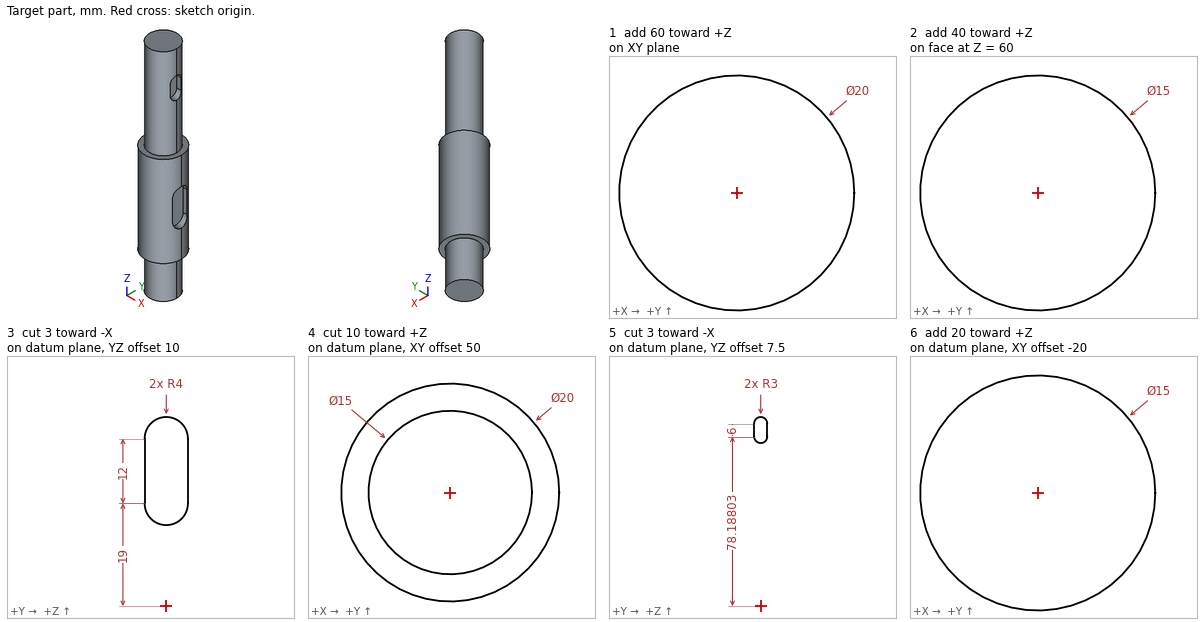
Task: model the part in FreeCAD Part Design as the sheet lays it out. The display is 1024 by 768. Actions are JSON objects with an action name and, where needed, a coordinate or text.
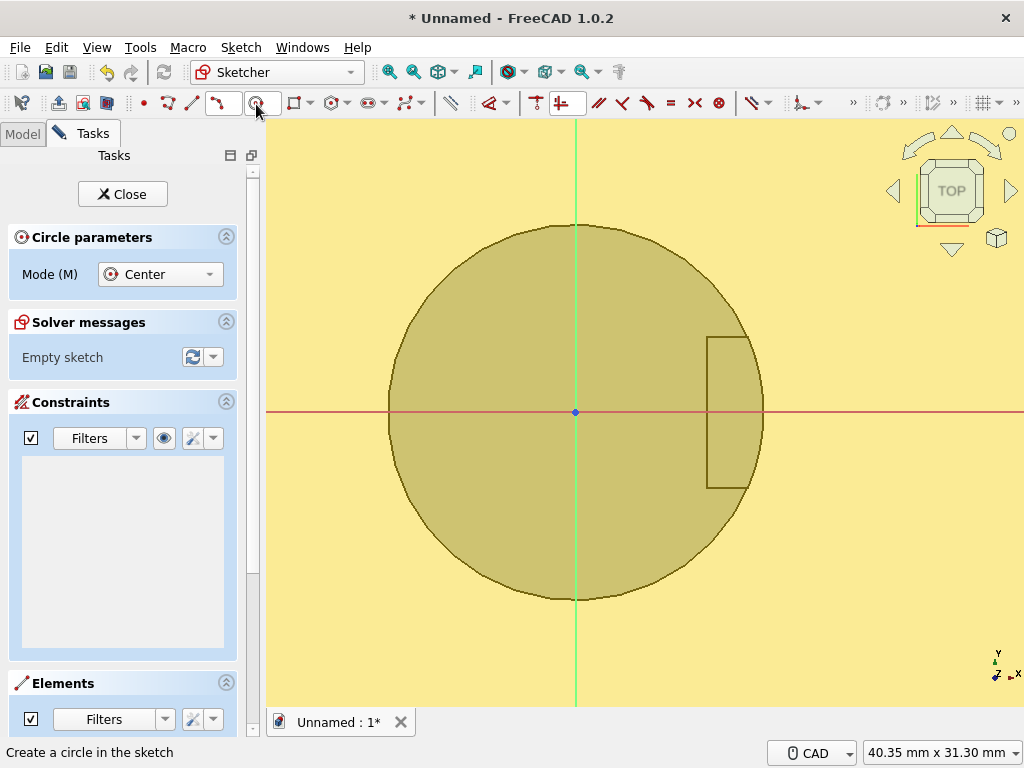
{"action": "left_click", "coordinate": [576, 412]}
{"action": "mouse_move", "coordinate": [708, 280]}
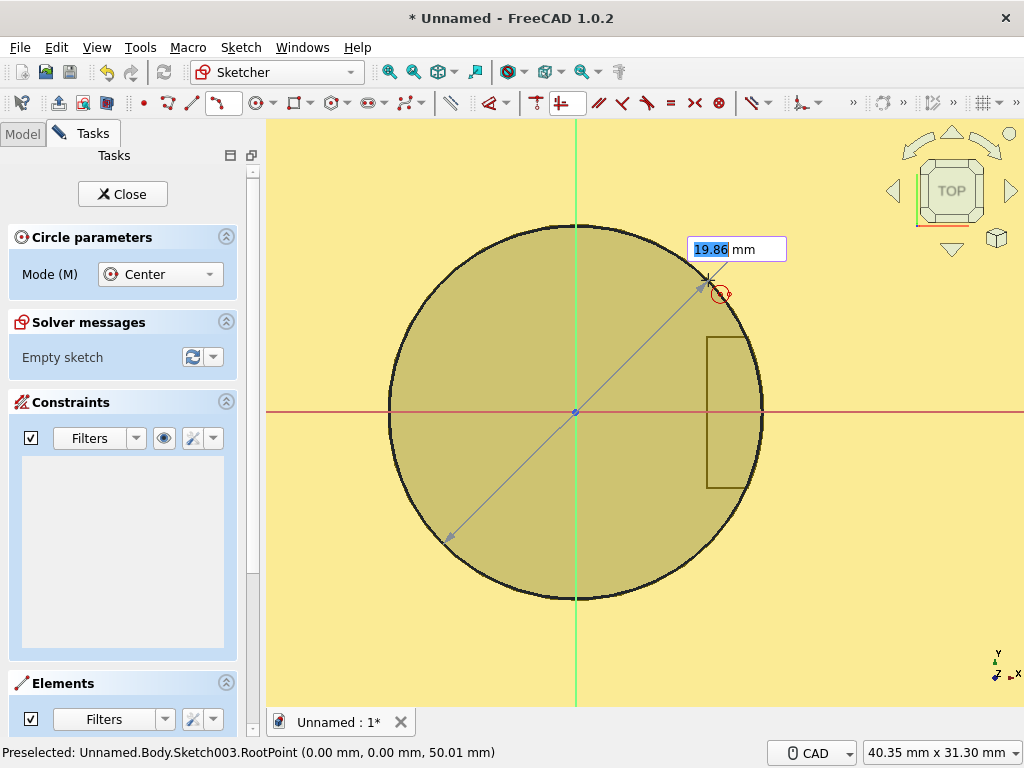
{"action": "type", "text": "20"}
{"action": "key", "text": "Return"}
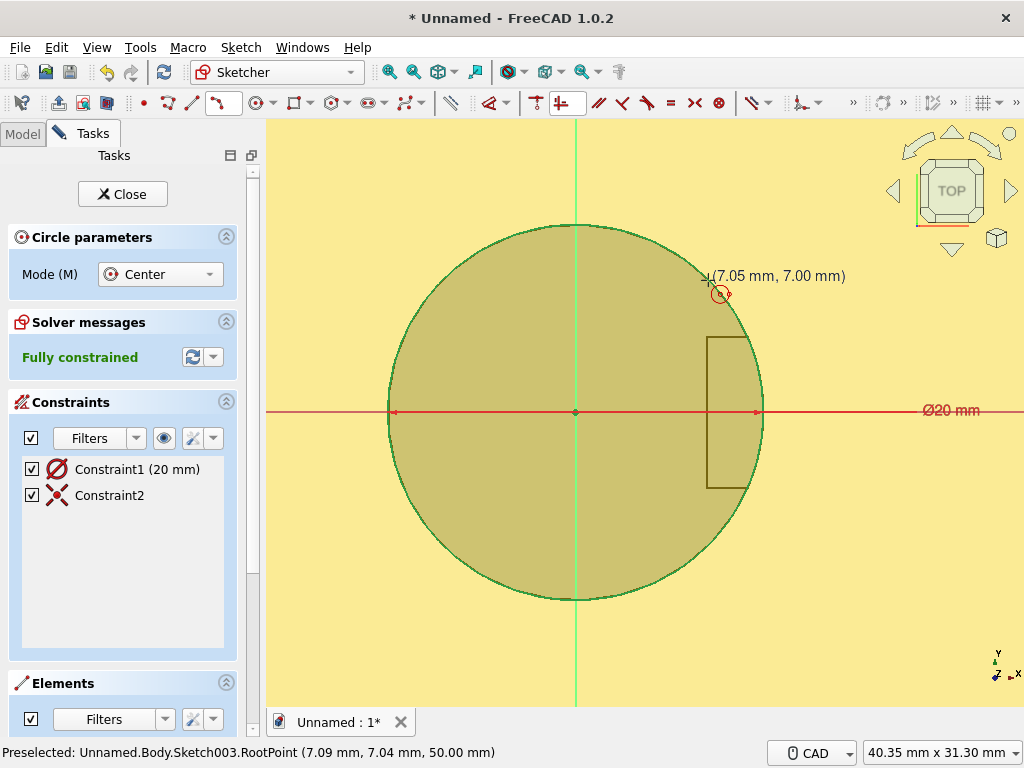
{"action": "left_click", "coordinate": [576, 412]}
{"action": "mouse_move", "coordinate": [675, 313]}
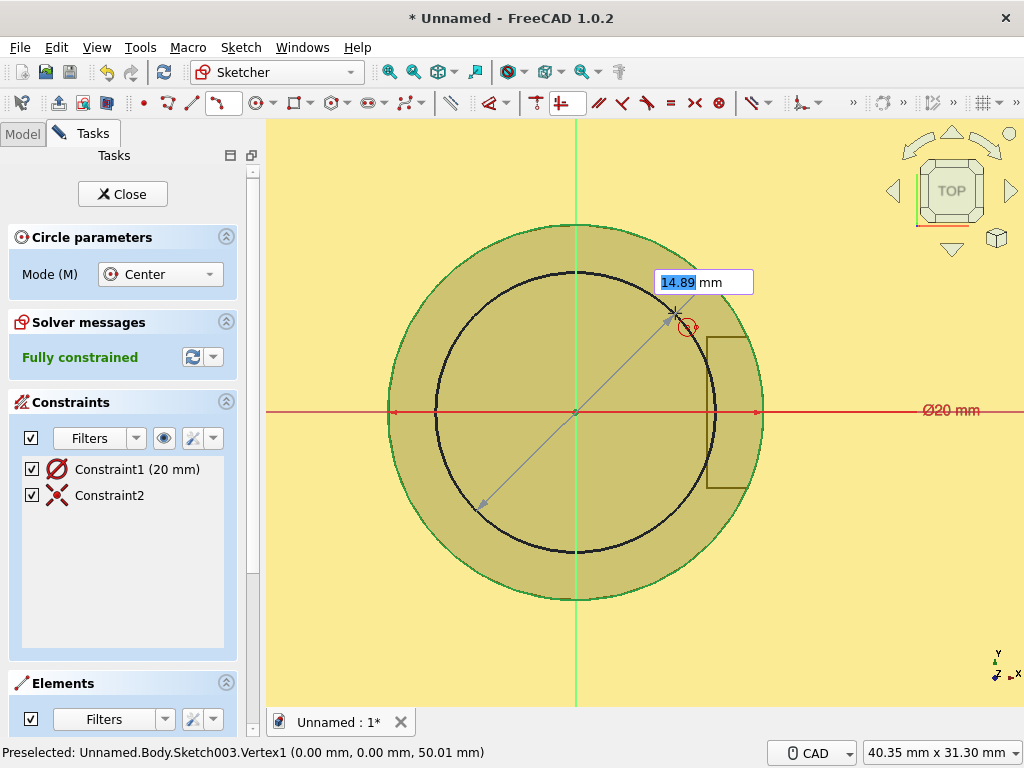
{"action": "type", "text": "15"}
{"action": "key", "text": "Return"}
{"action": "key", "text": "Escape"}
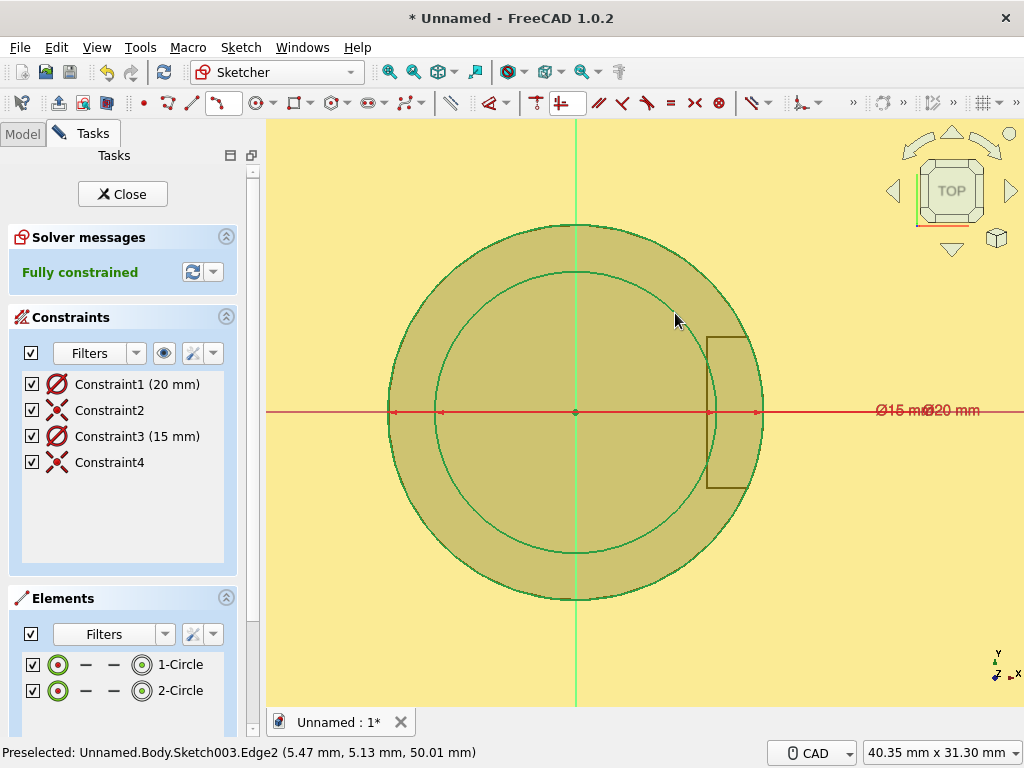
{"action": "left_click", "coordinate": [123, 194]}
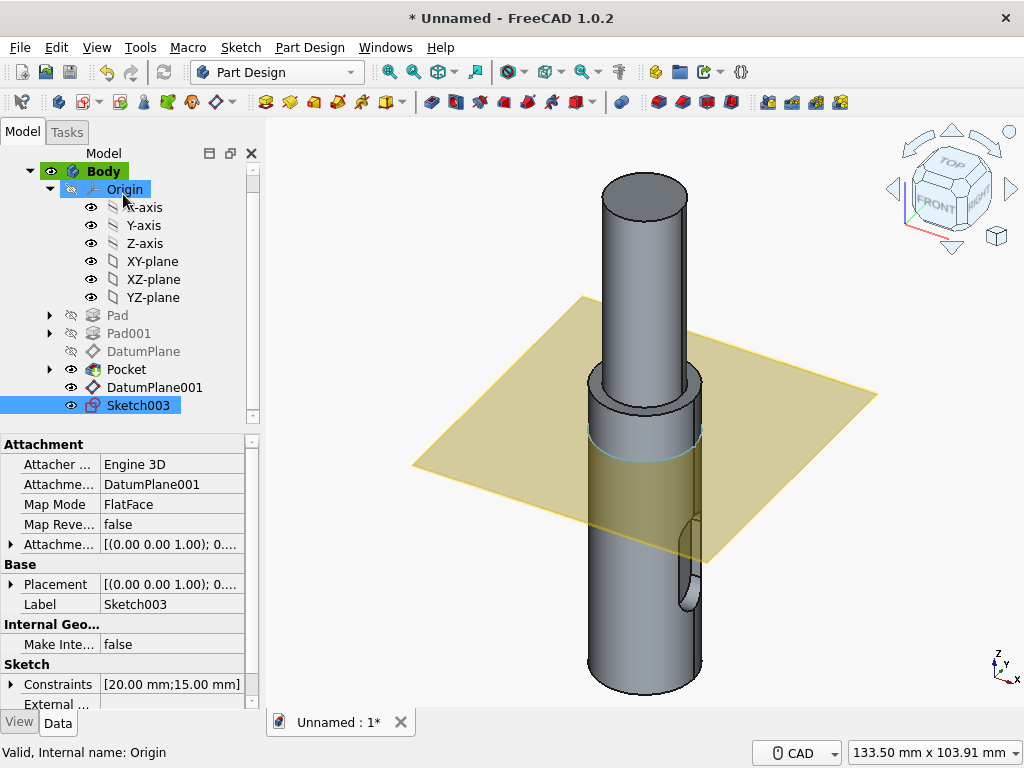
{"action": "left_click", "coordinate": [432, 102]}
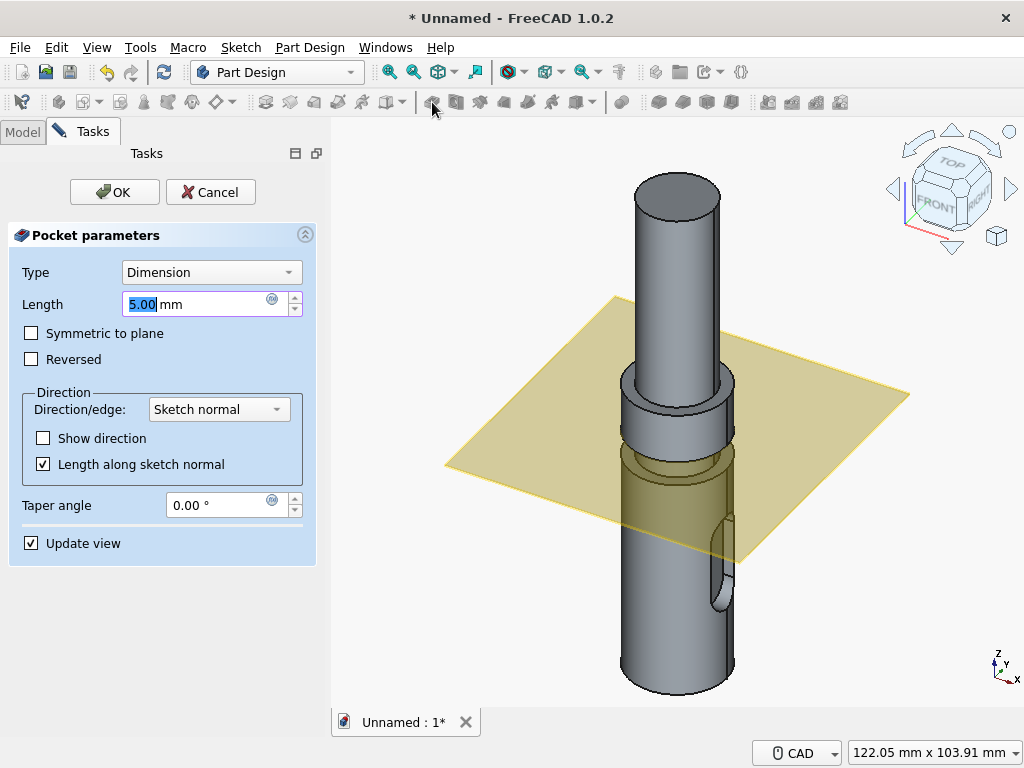
{"action": "type", "text": "10"}
{"action": "key", "text": "Tab"}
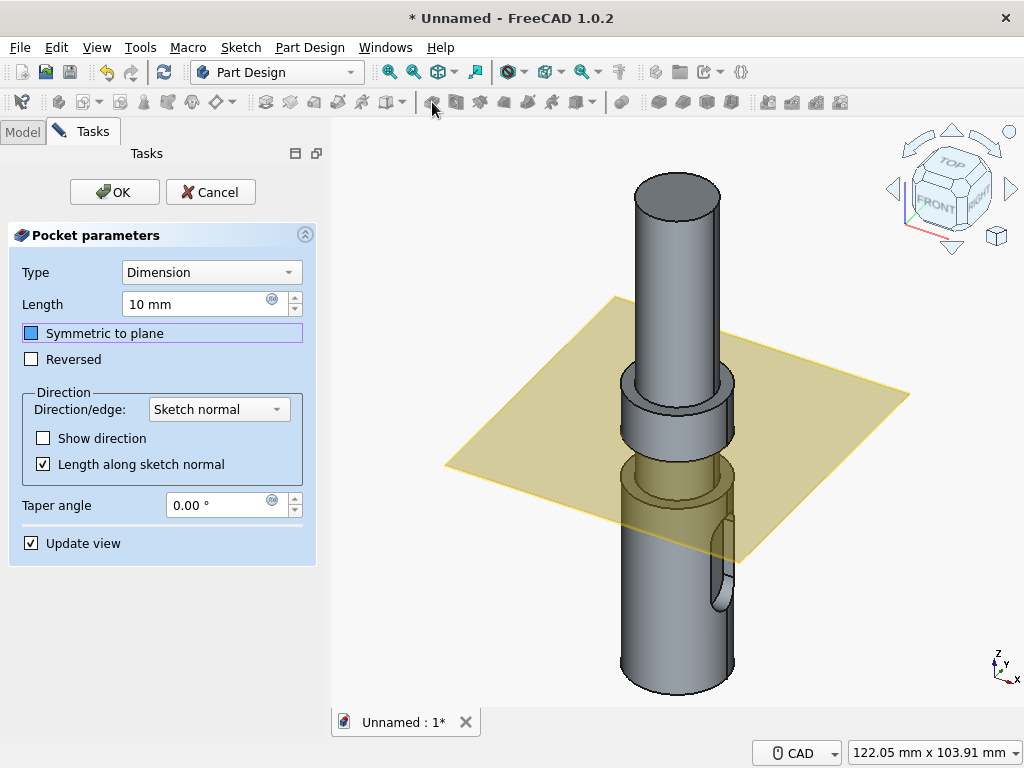
{"action": "left_click", "coordinate": [30, 359]}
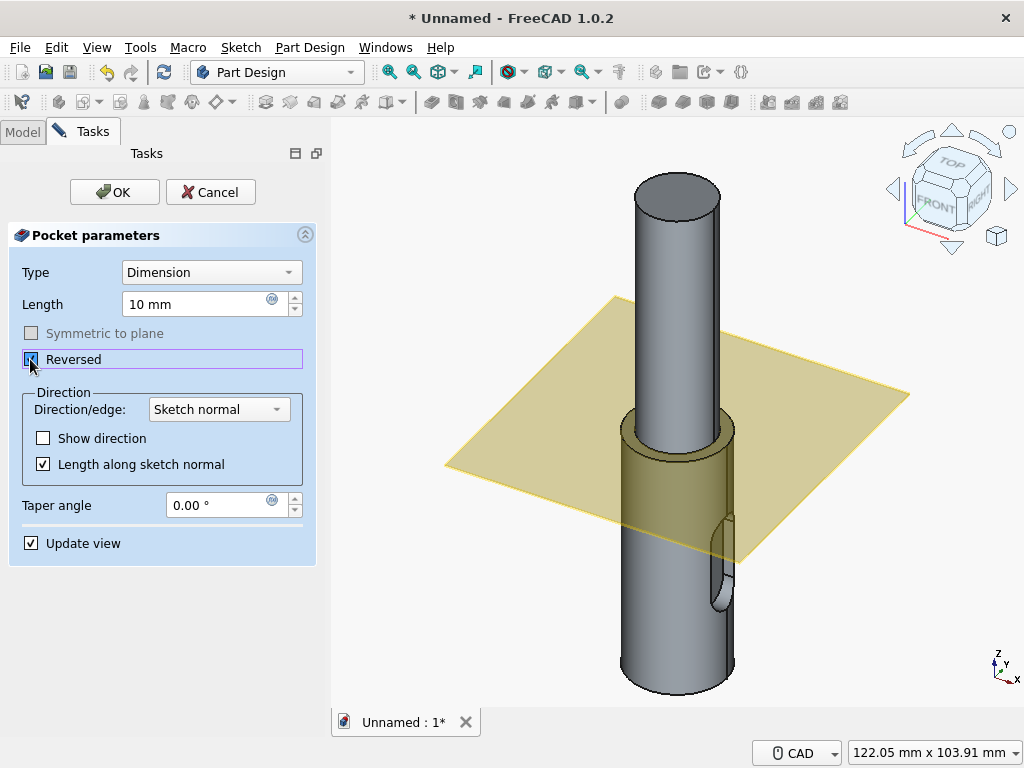
{"action": "left_click", "coordinate": [115, 192]}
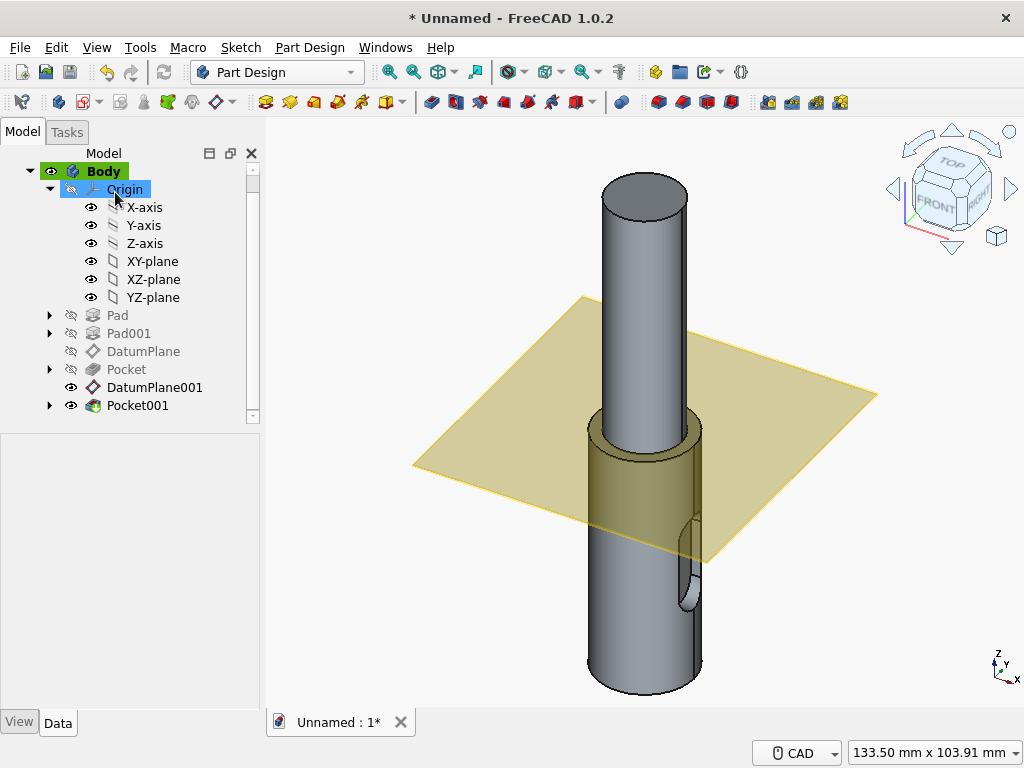
{"action": "left_click", "coordinate": [116, 387]}
{"action": "key", "text": "space"}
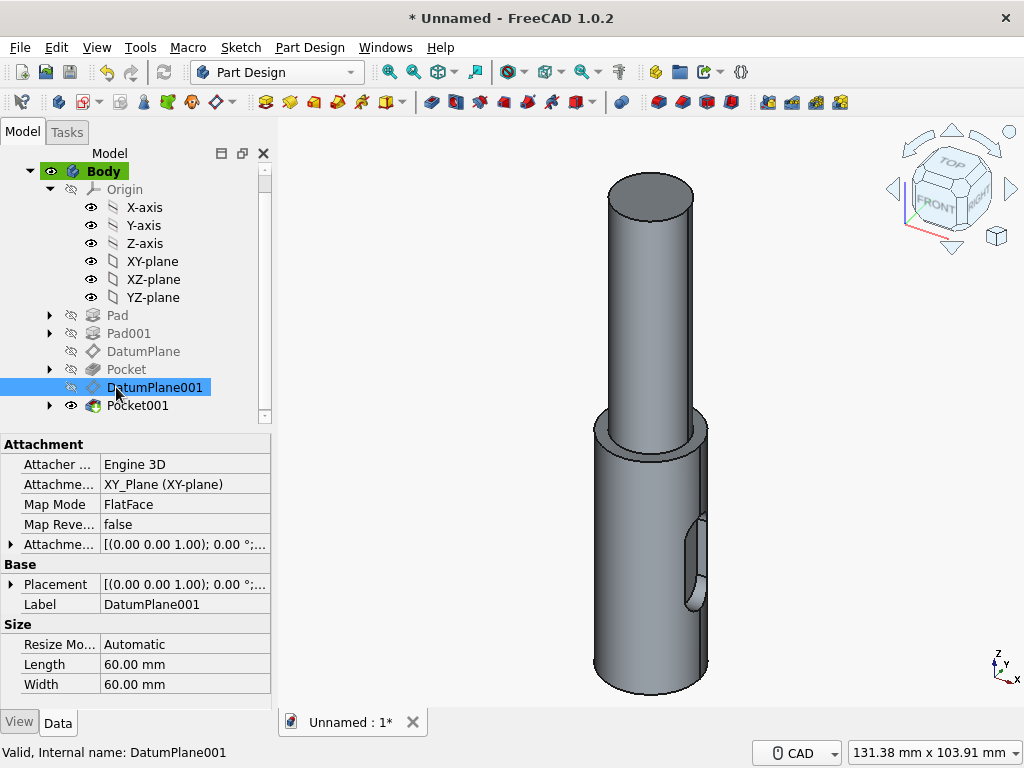
{"action": "left_click", "coordinate": [136, 297]}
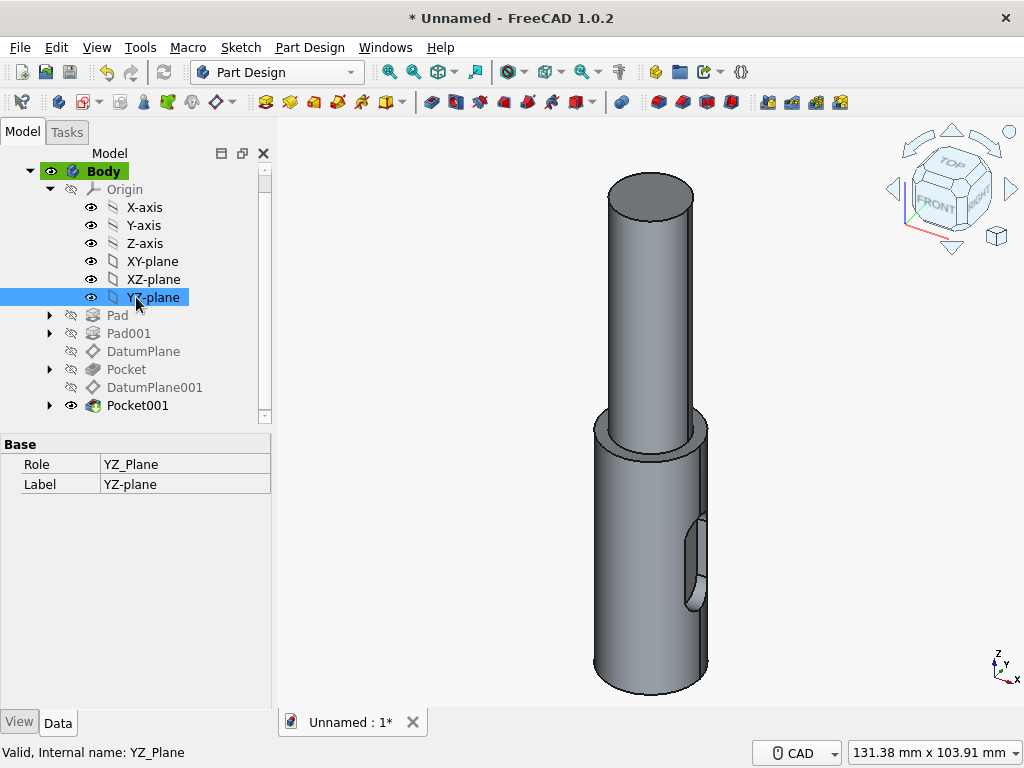
{"action": "left_click", "coordinate": [216, 102]}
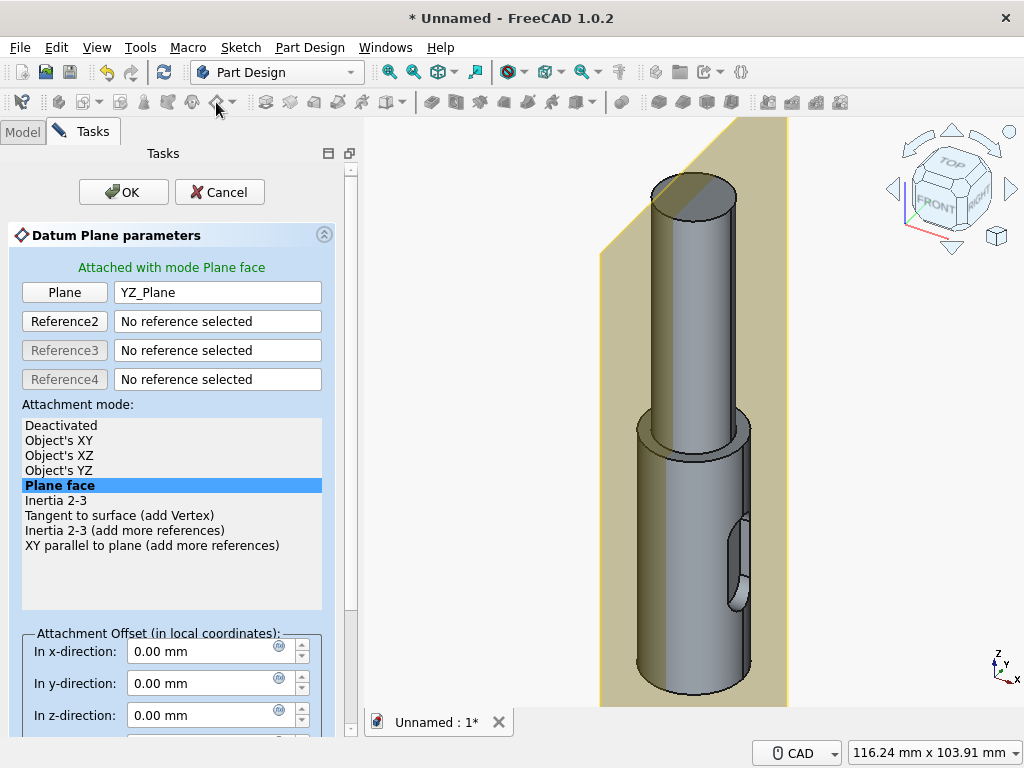
{"action": "triple_click", "coordinate": [210, 715]}